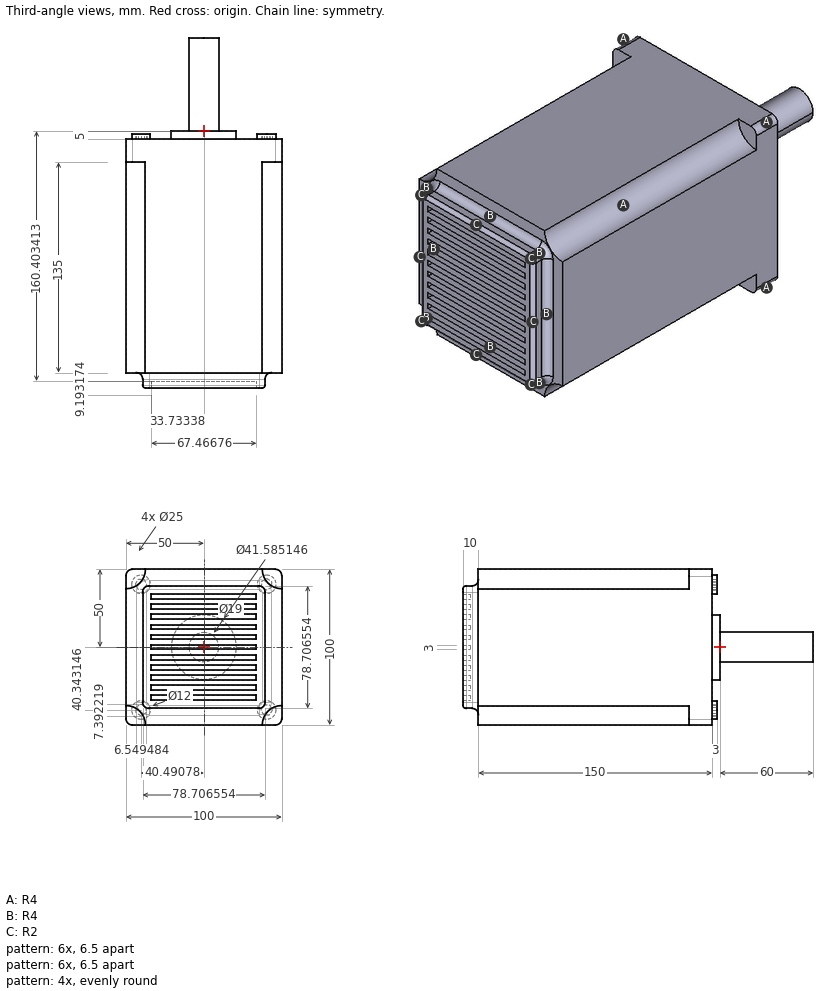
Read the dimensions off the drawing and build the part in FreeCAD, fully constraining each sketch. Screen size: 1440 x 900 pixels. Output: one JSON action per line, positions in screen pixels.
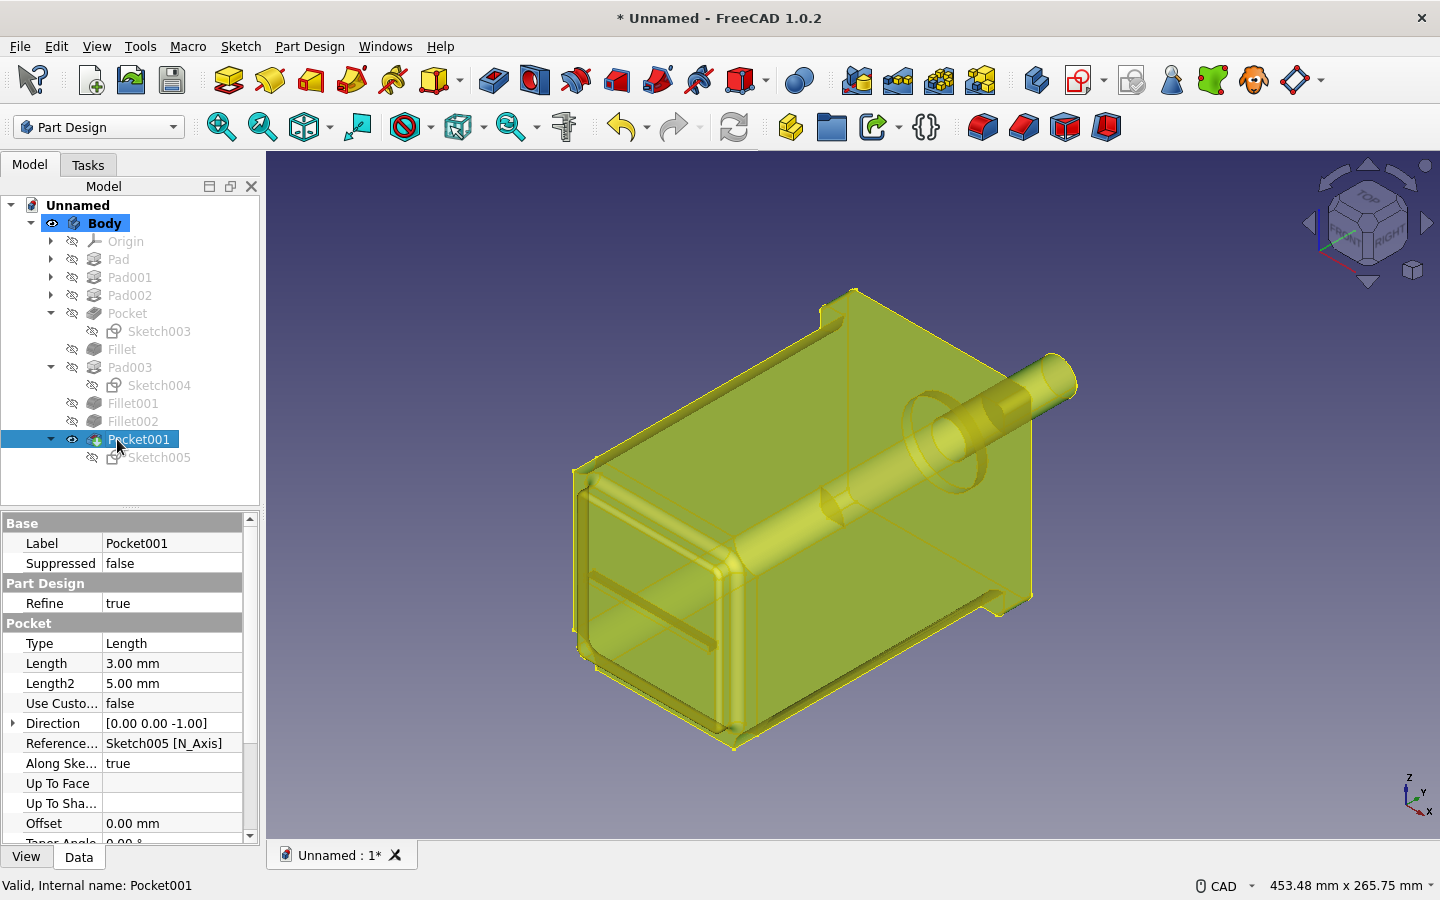
{"action": "left_click", "coordinate": [898, 80]}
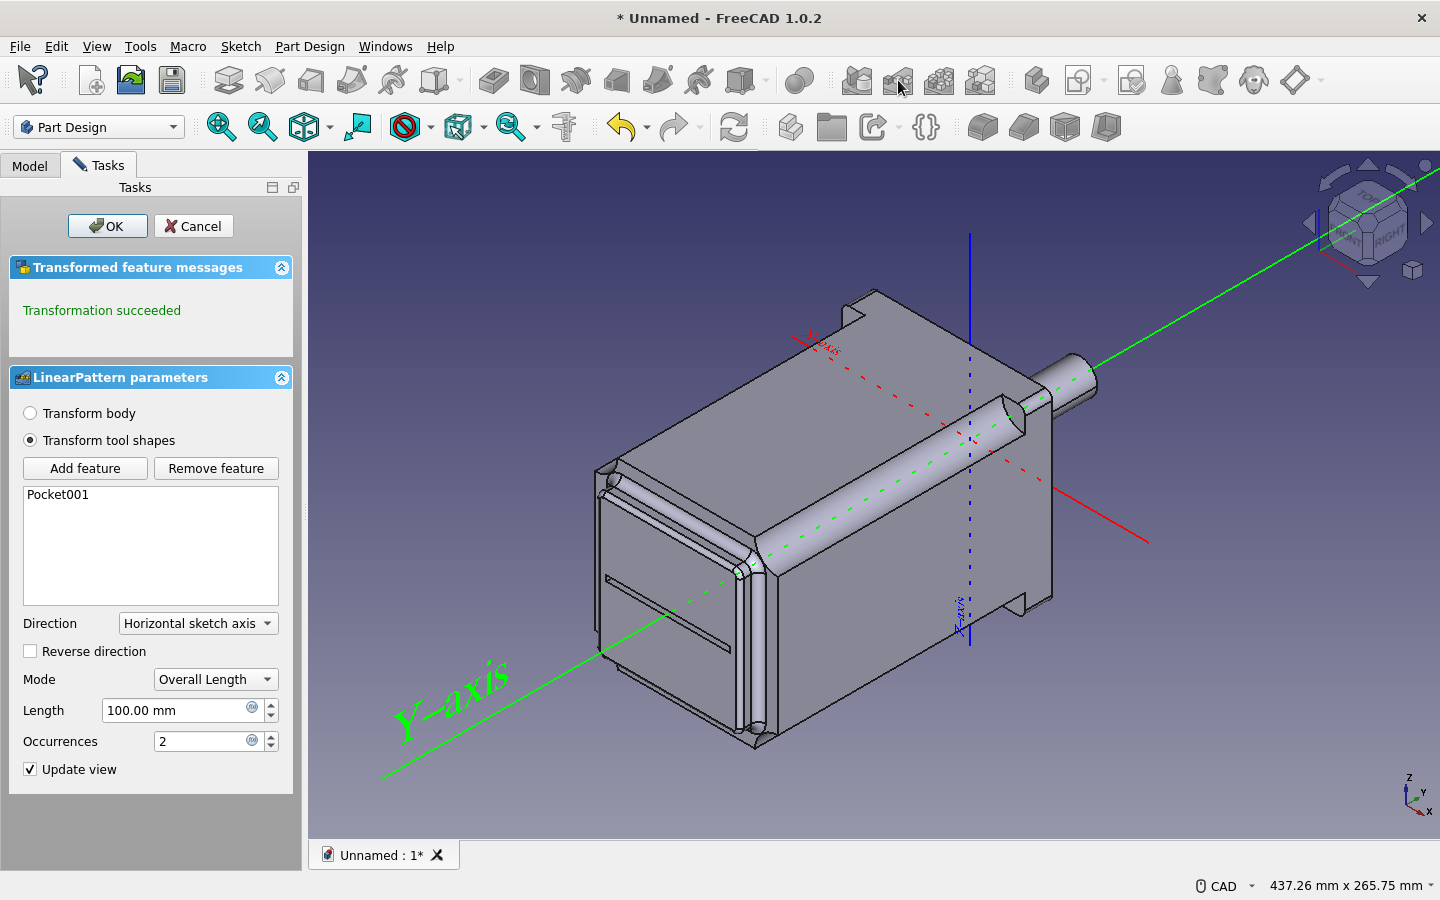
{"action": "left_click", "coordinate": [199, 624]}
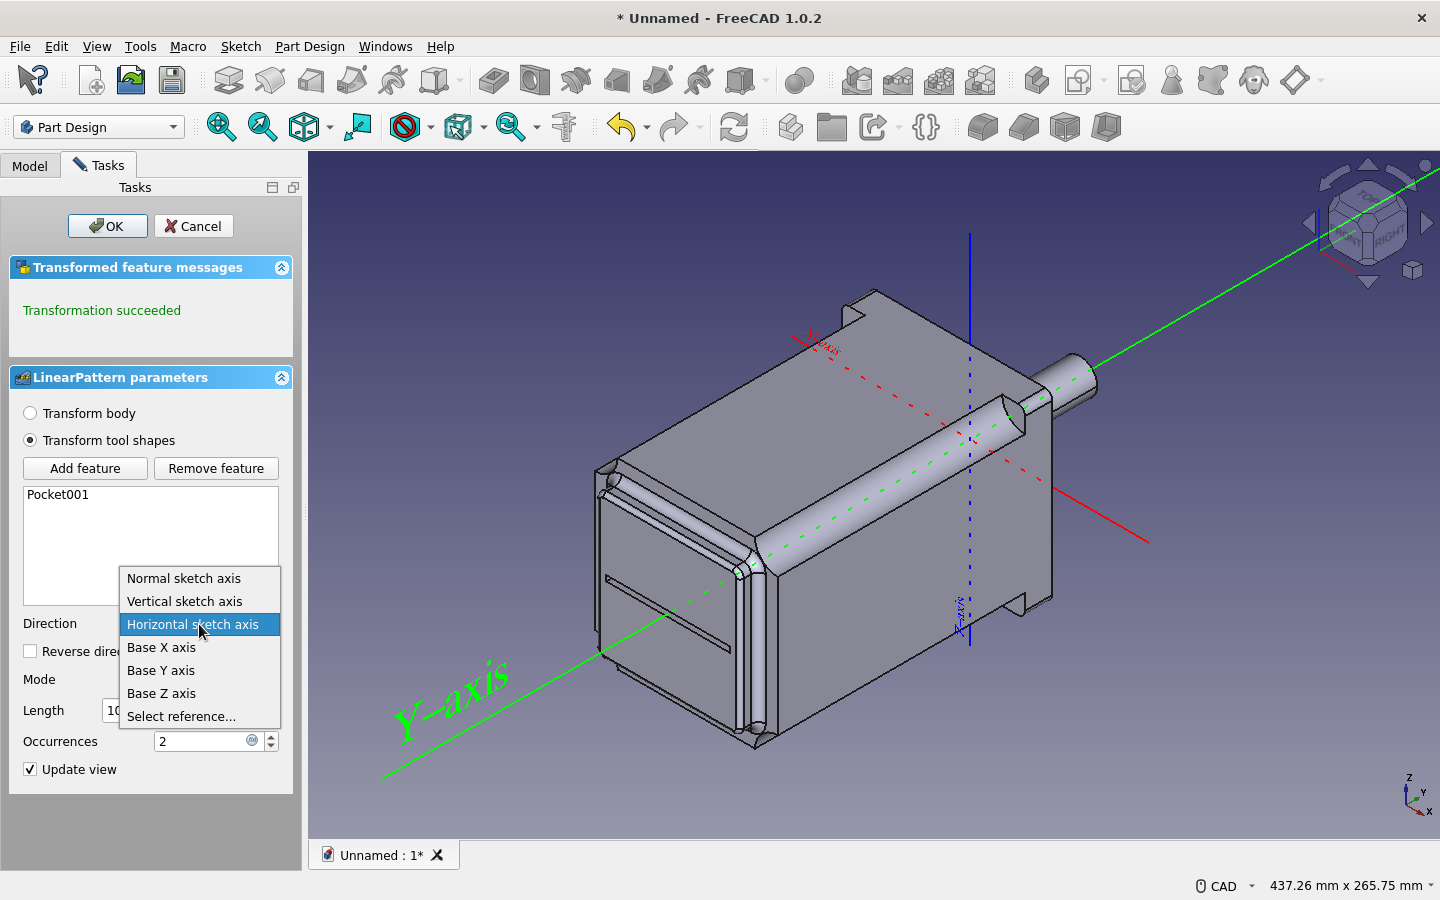
{"action": "left_click", "coordinate": [198, 694]}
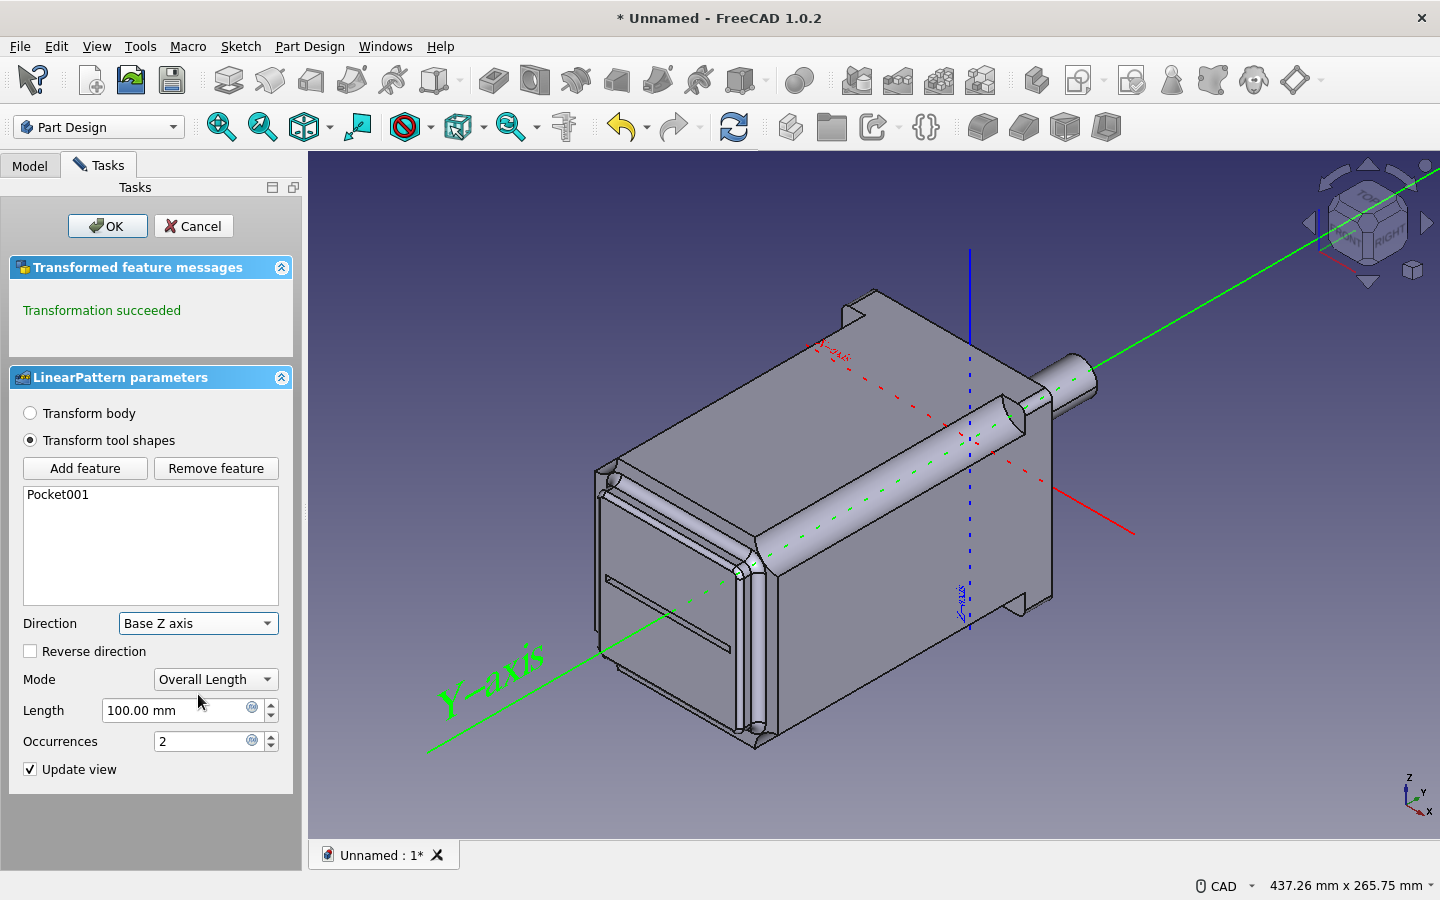
{"action": "left_click", "coordinate": [216, 680]}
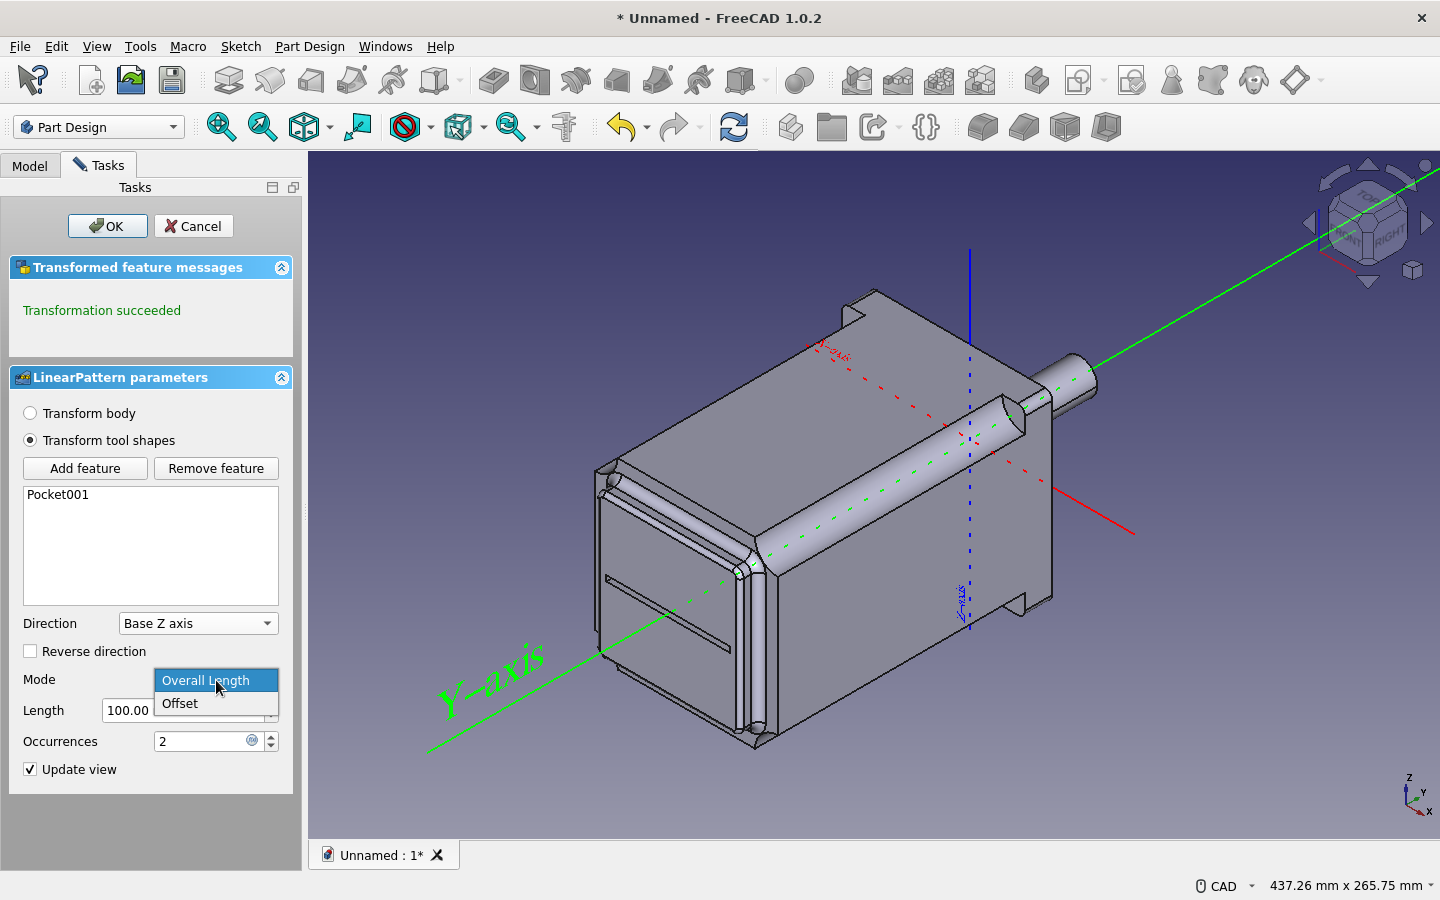
{"action": "left_click", "coordinate": [214, 704]}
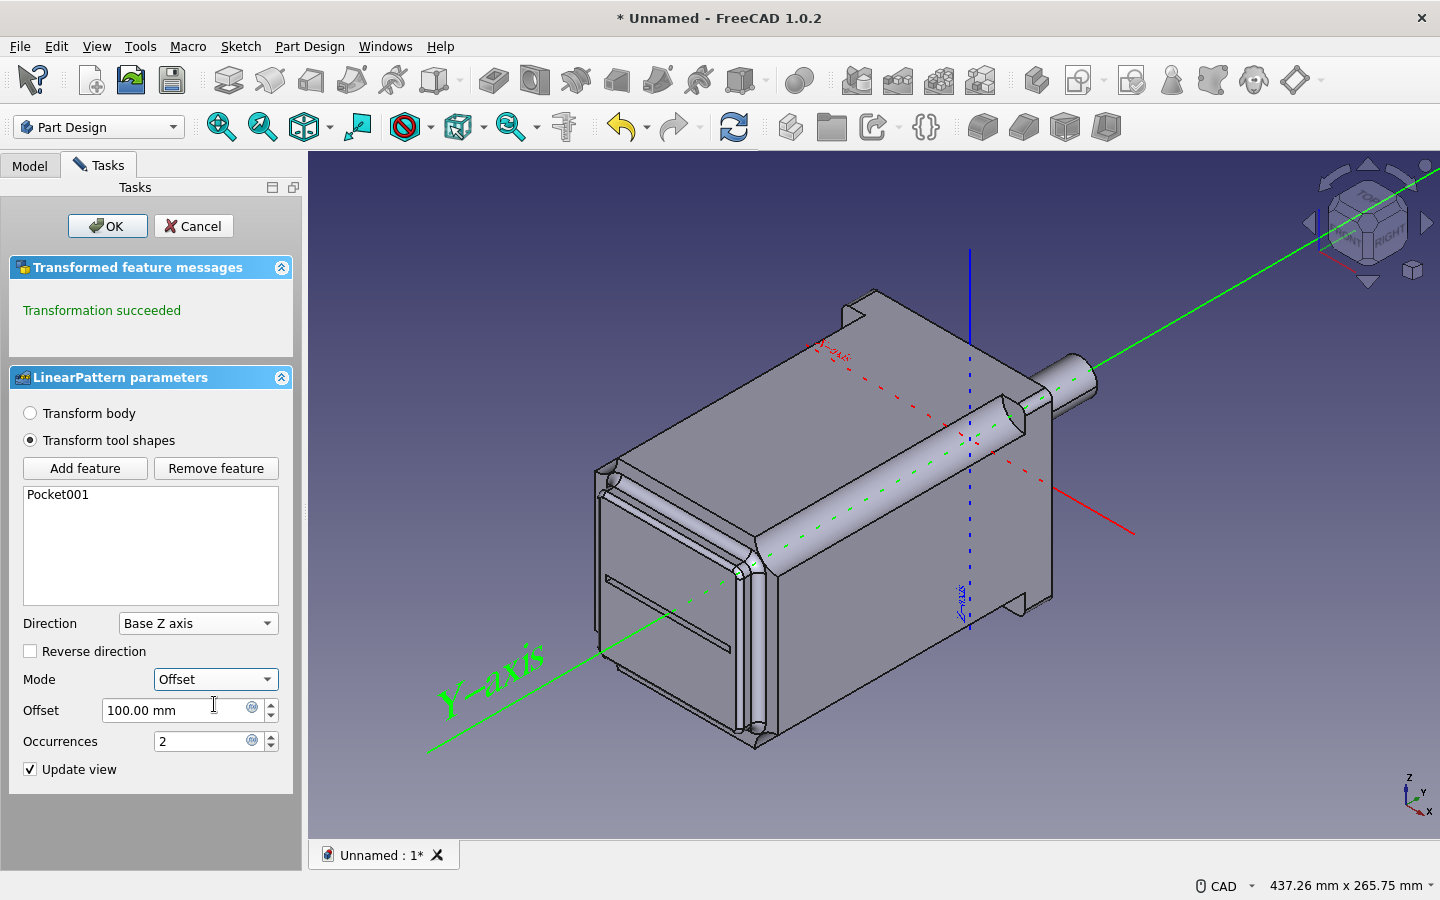
{"action": "triple_click", "coordinate": [184, 710]}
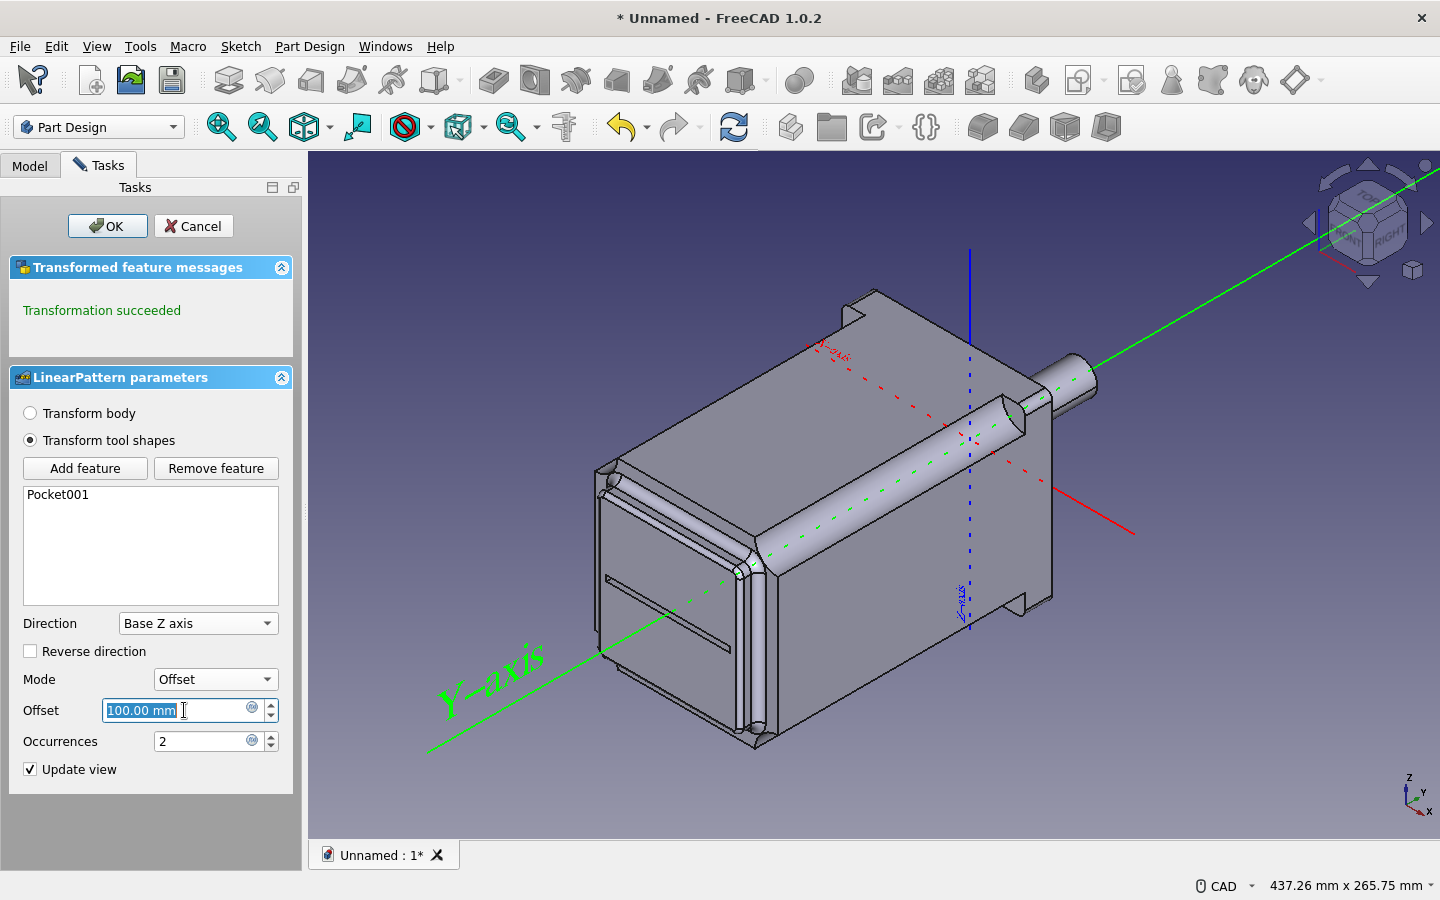
{"action": "type", "text": "6.5"}
{"action": "key", "text": "Tab"}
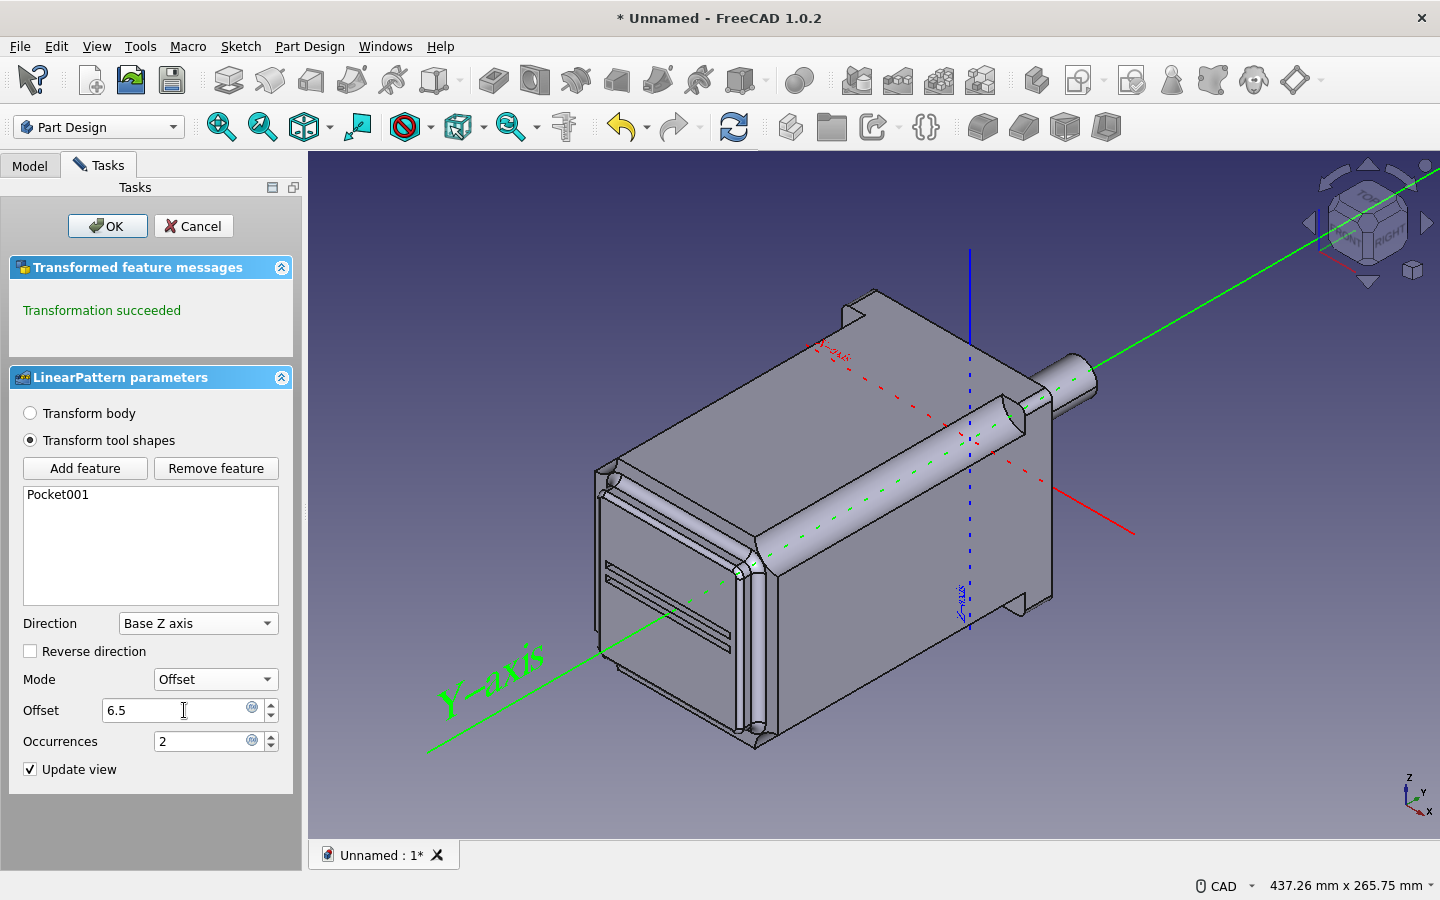
{"action": "triple_click", "coordinate": [210, 742]}